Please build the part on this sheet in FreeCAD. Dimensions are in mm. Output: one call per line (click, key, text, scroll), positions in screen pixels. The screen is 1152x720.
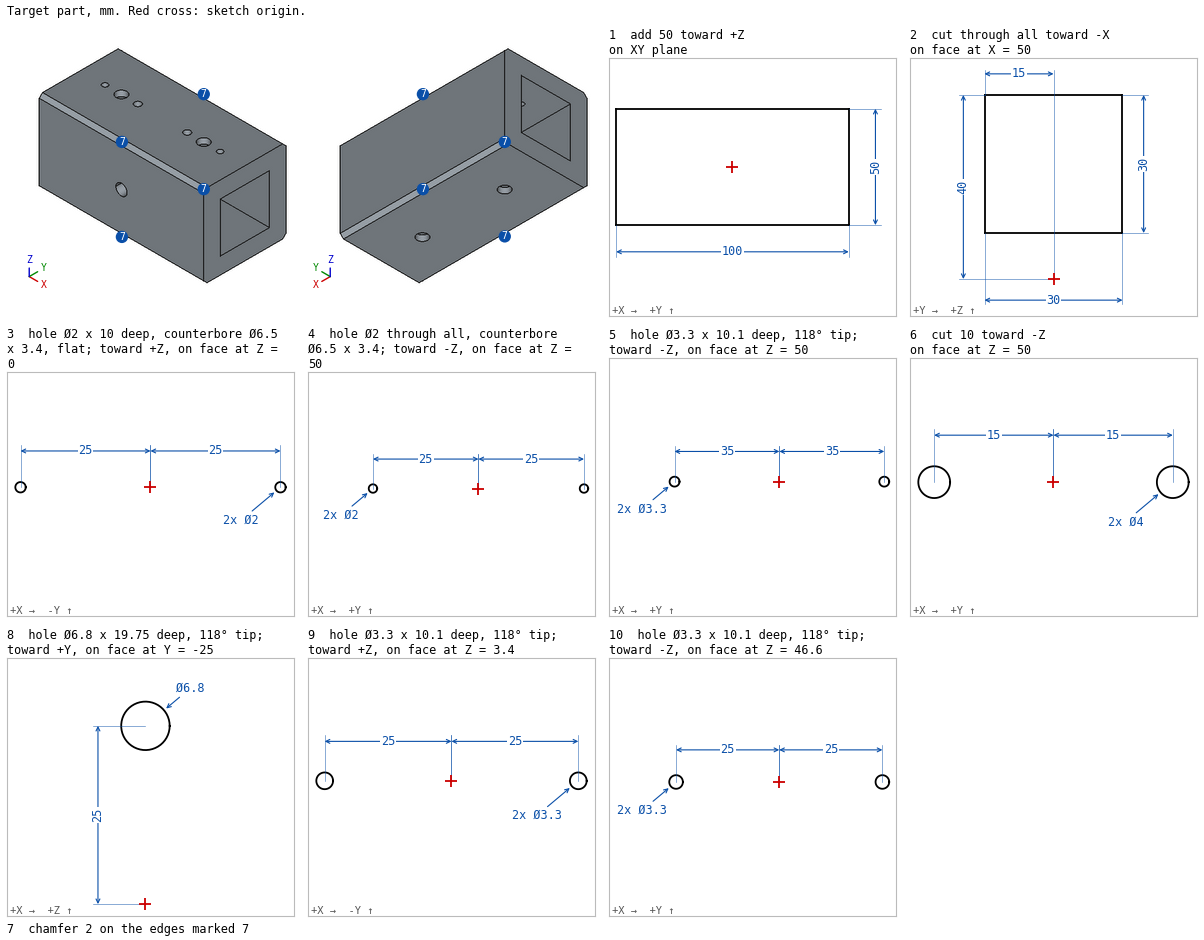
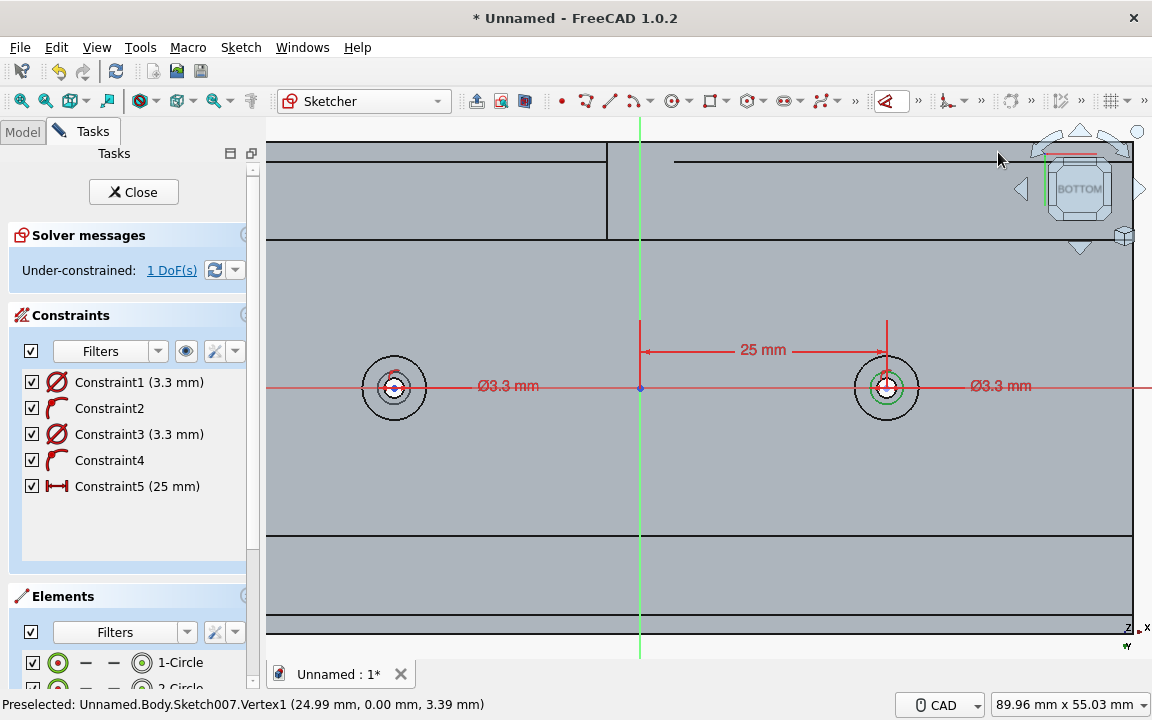
click(394, 388)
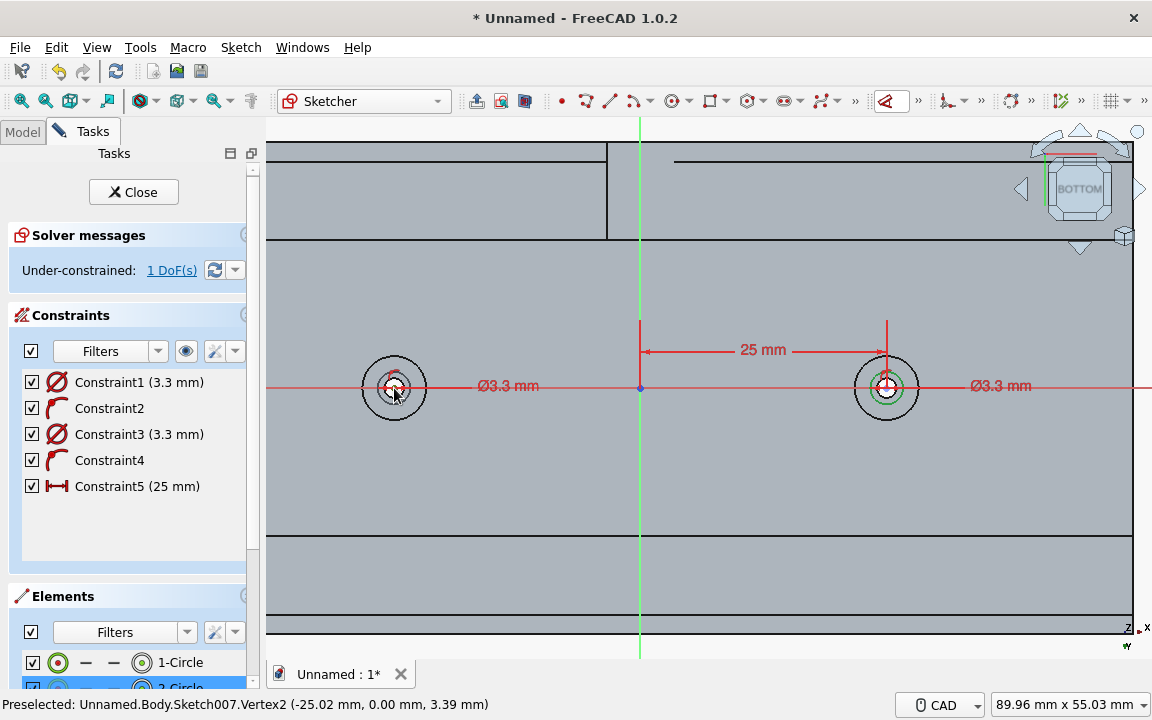
click(904, 102)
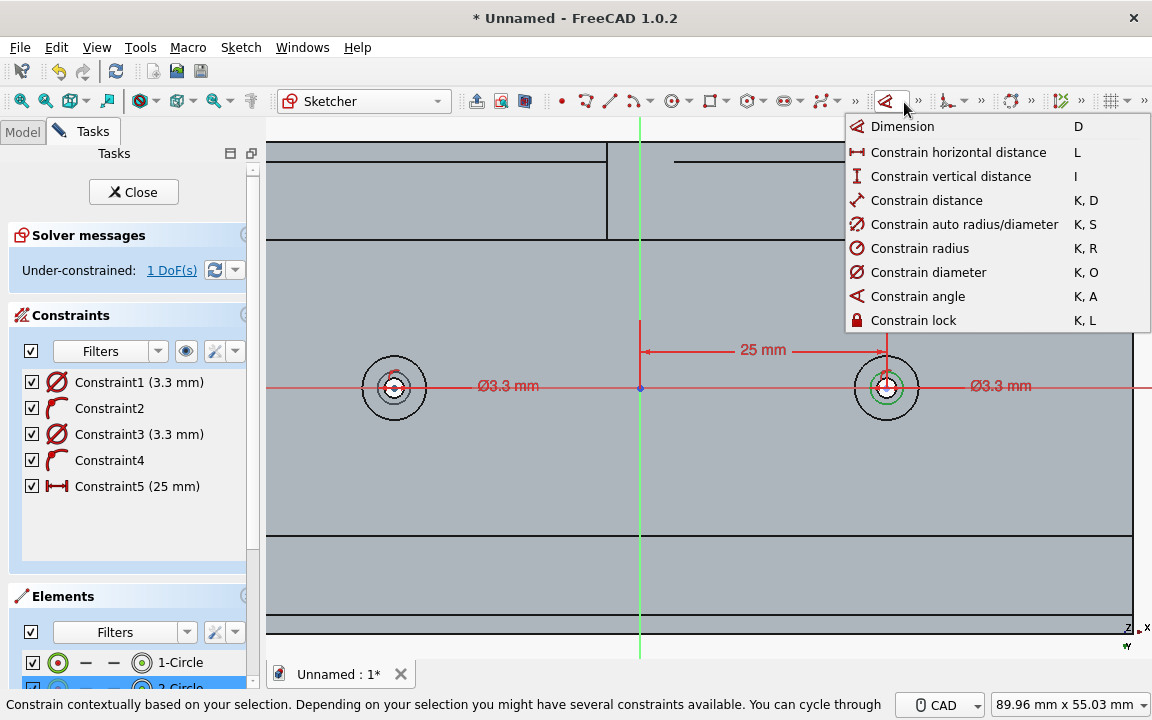
click(998, 152)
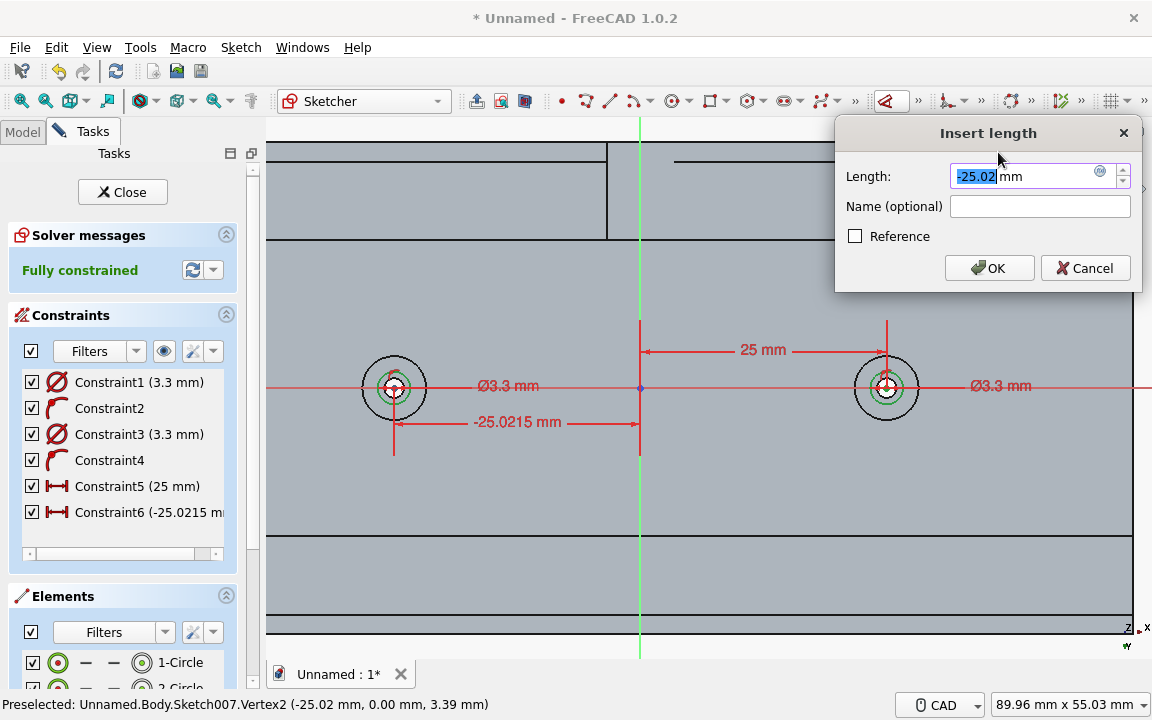
text(-25)
key(Return)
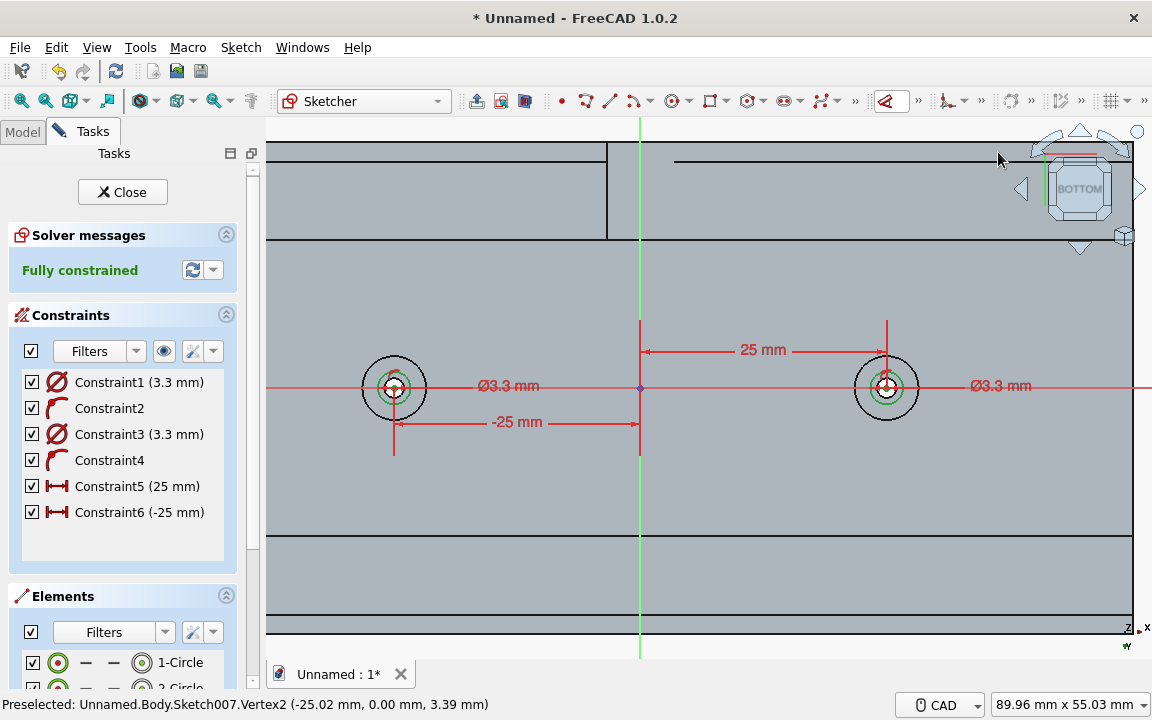
click(123, 192)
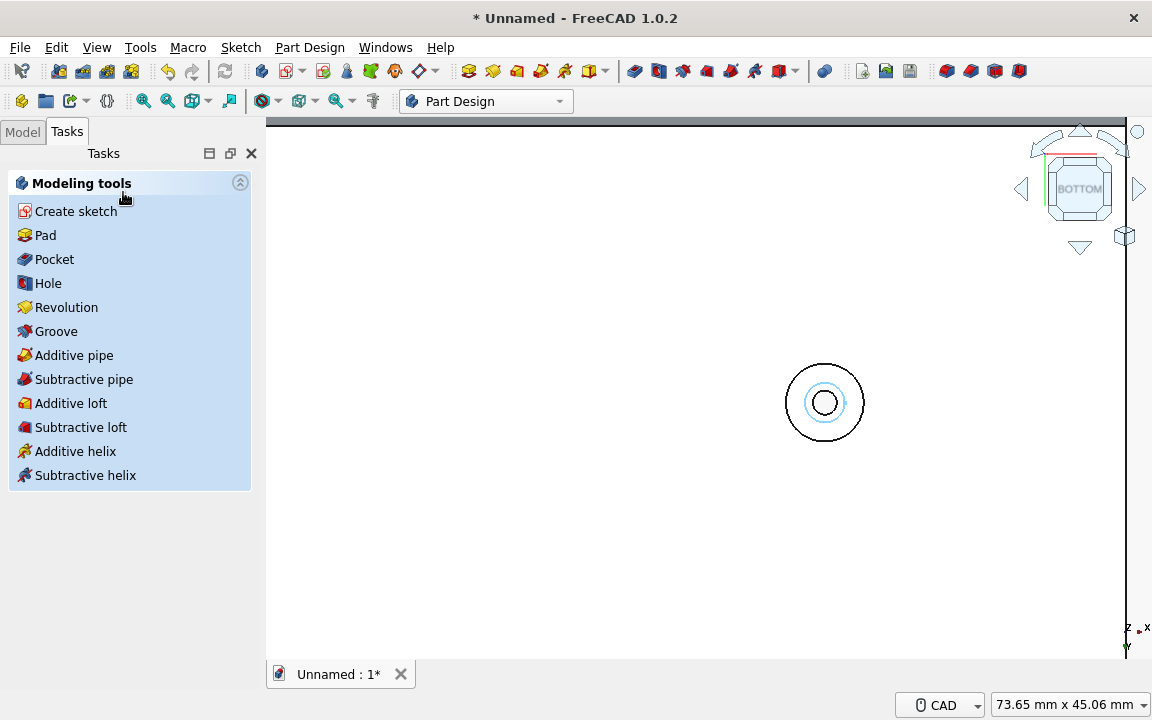
click(660, 72)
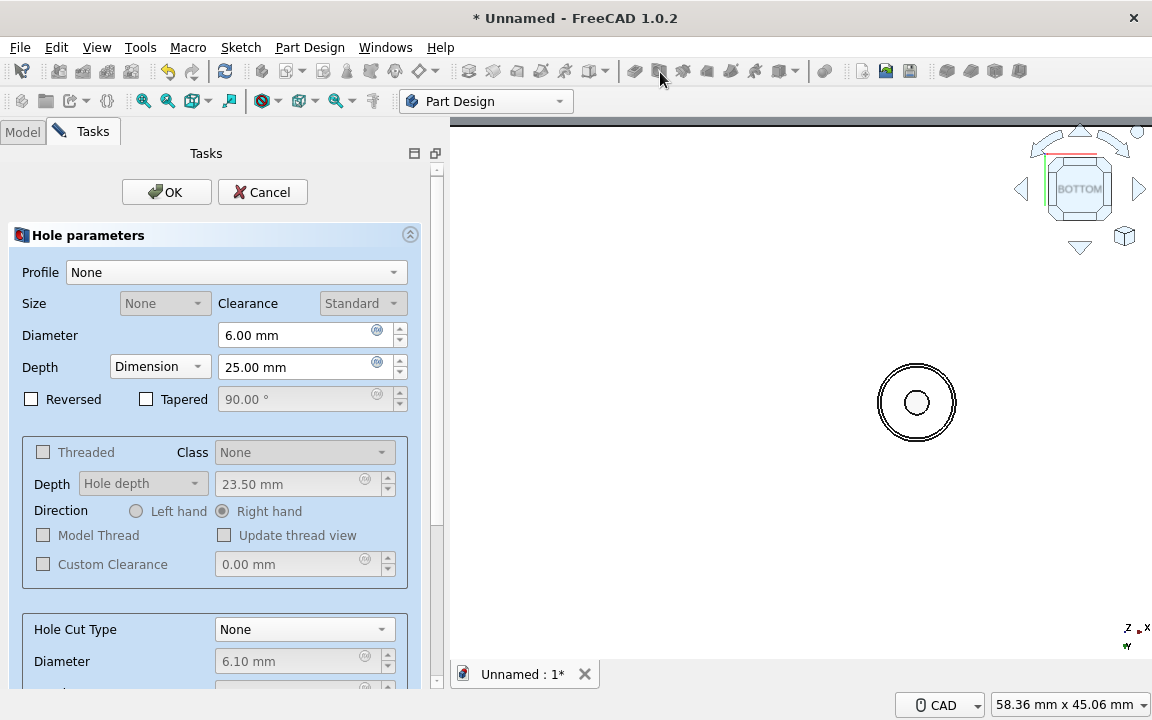
triple_click(305, 335)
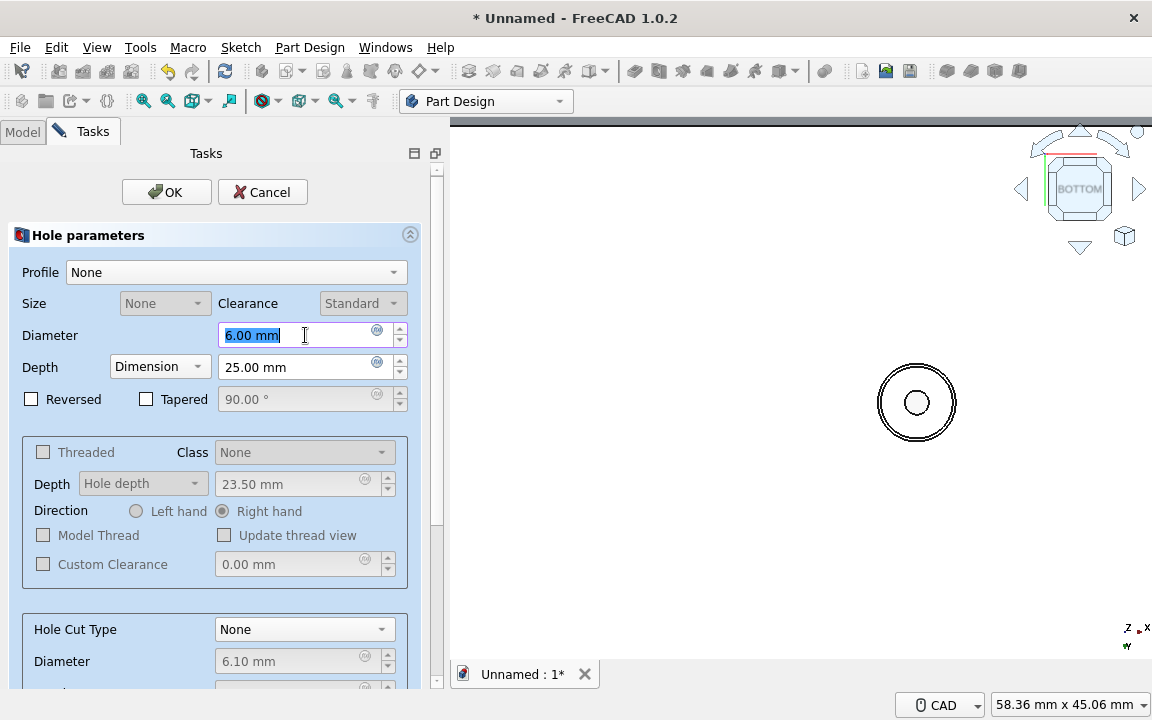
text(3.3)
key(Tab)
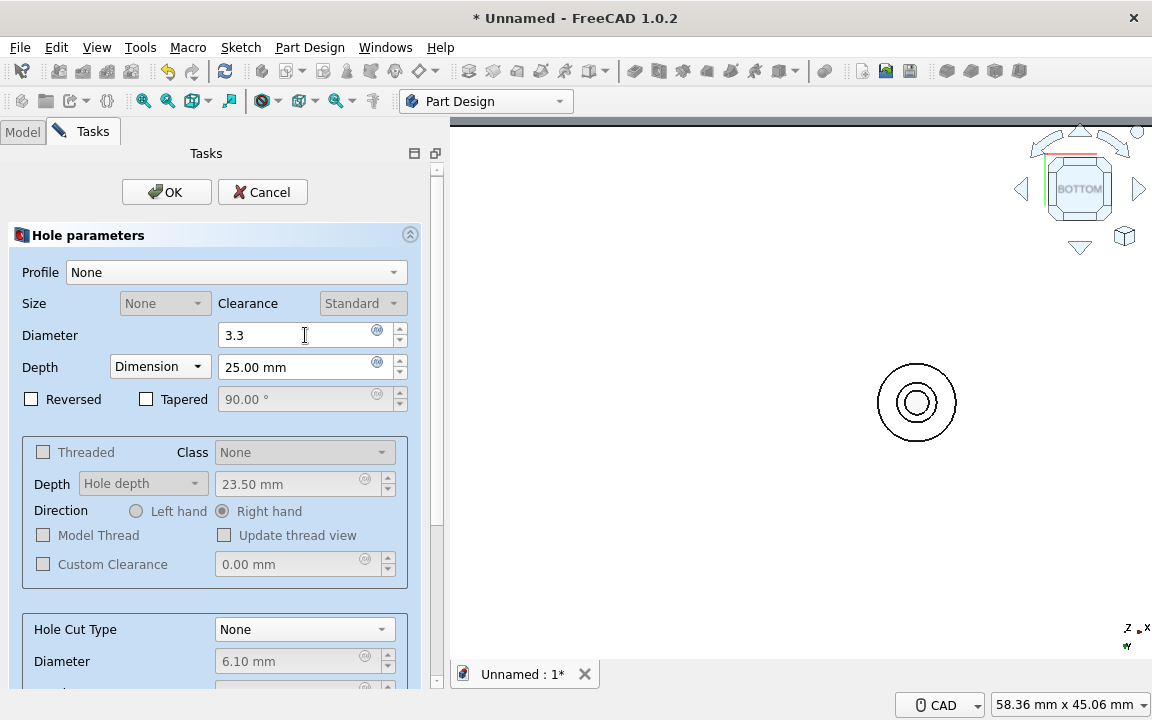
triple_click(305, 367)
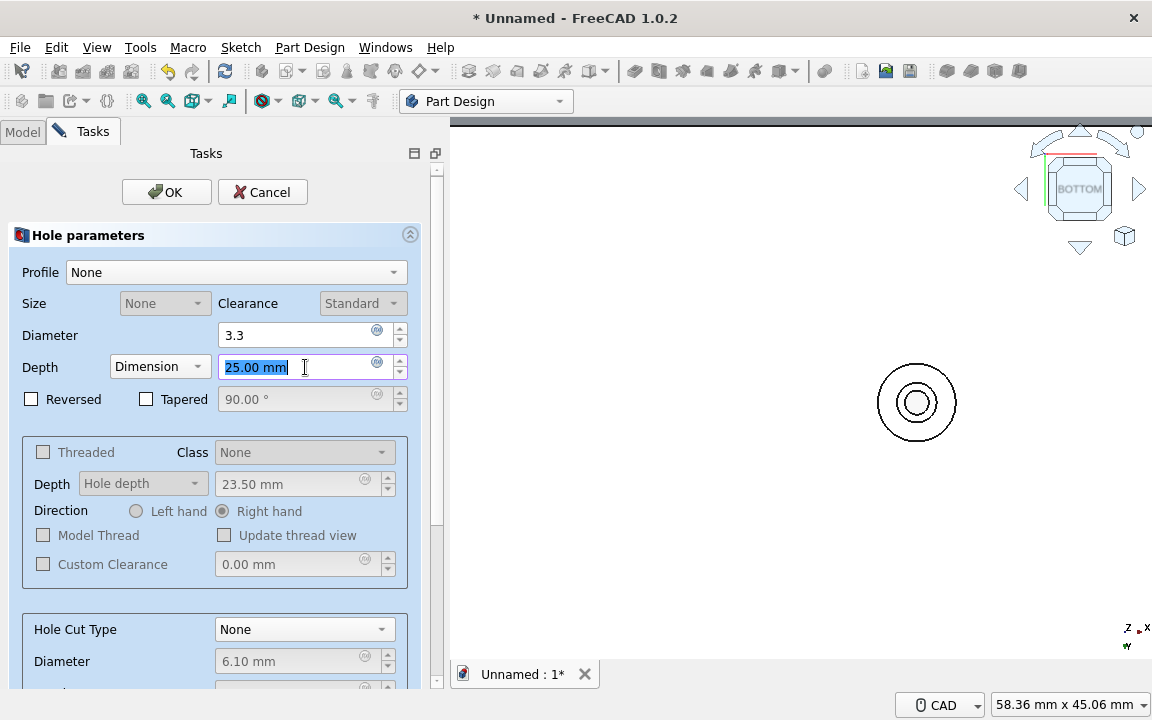
text(10.1)
key(Tab)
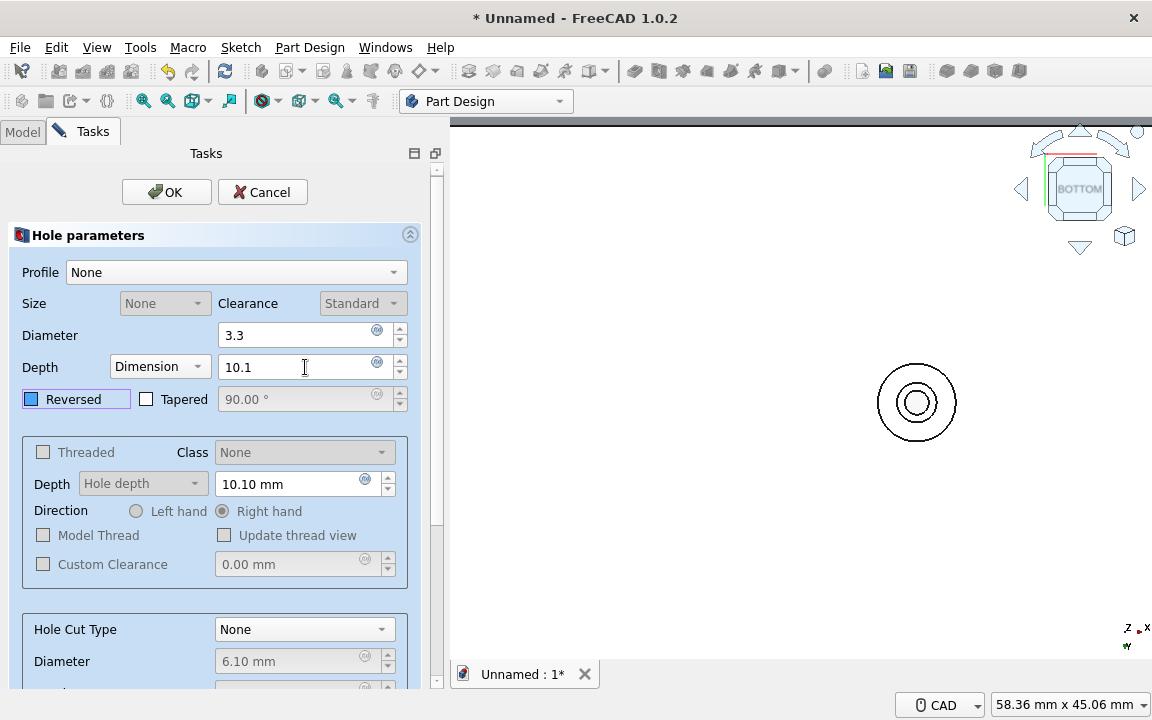
click(167, 192)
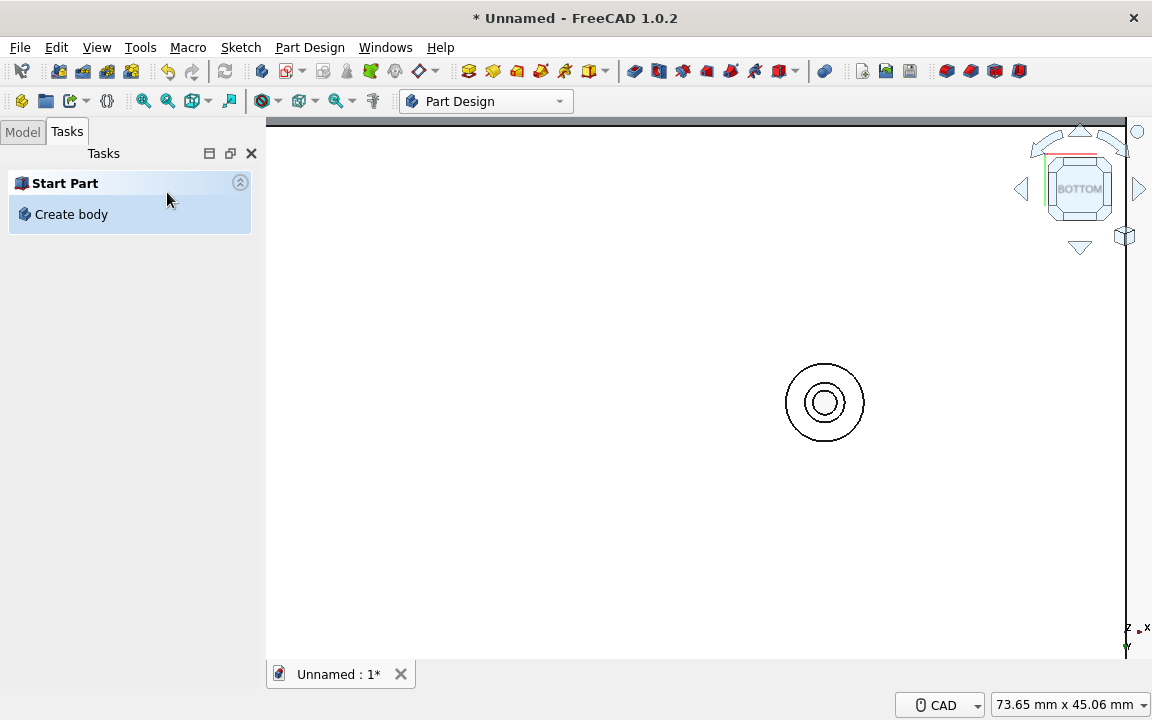
key(v)
key(f)